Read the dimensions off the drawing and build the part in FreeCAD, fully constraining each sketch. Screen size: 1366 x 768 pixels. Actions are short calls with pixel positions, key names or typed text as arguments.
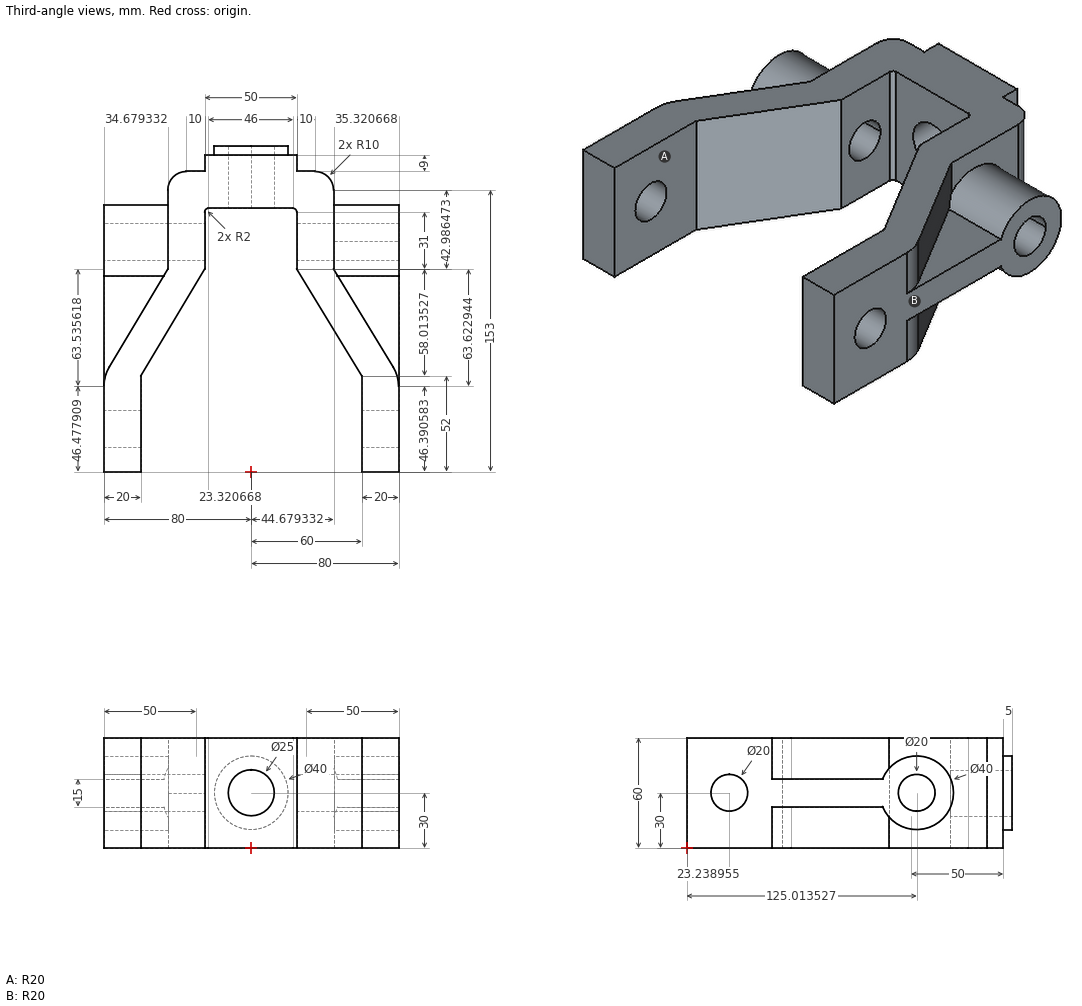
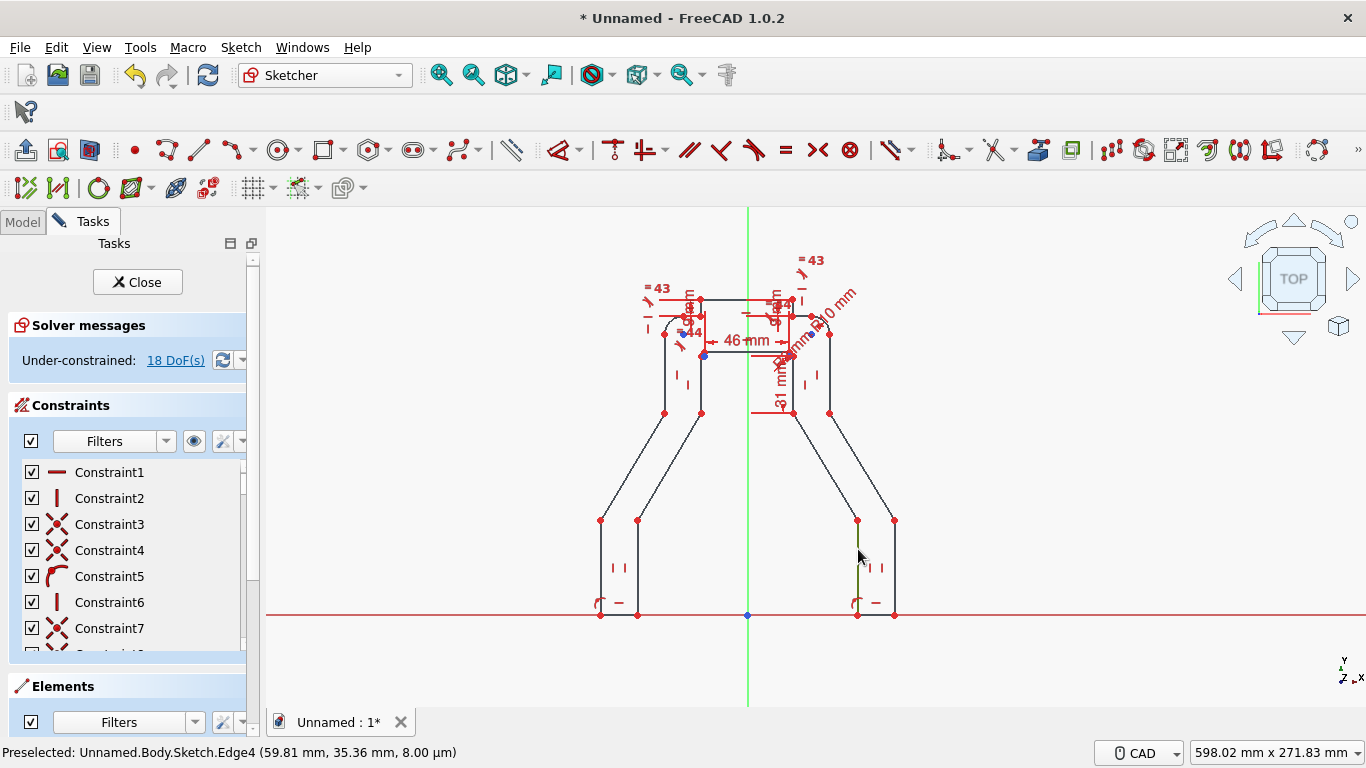
key(i)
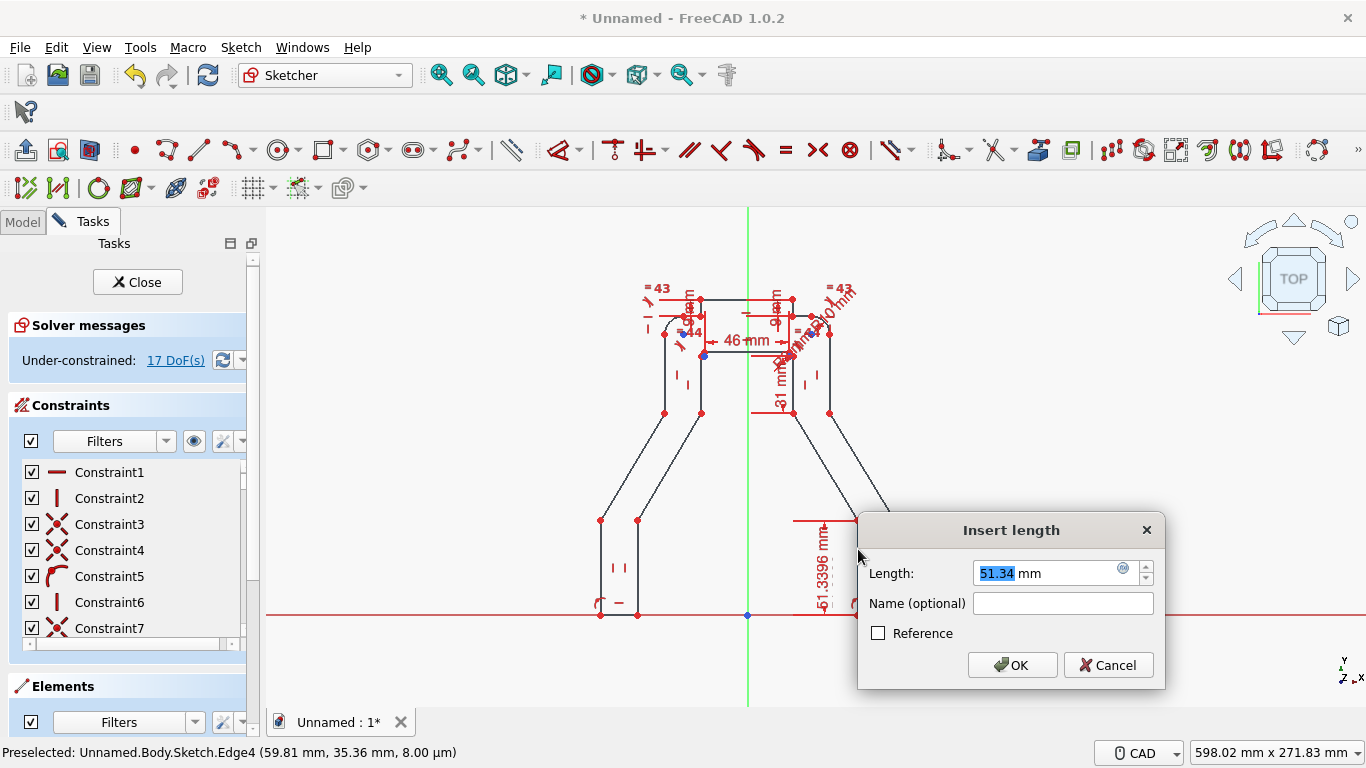
text(52)
key(Return)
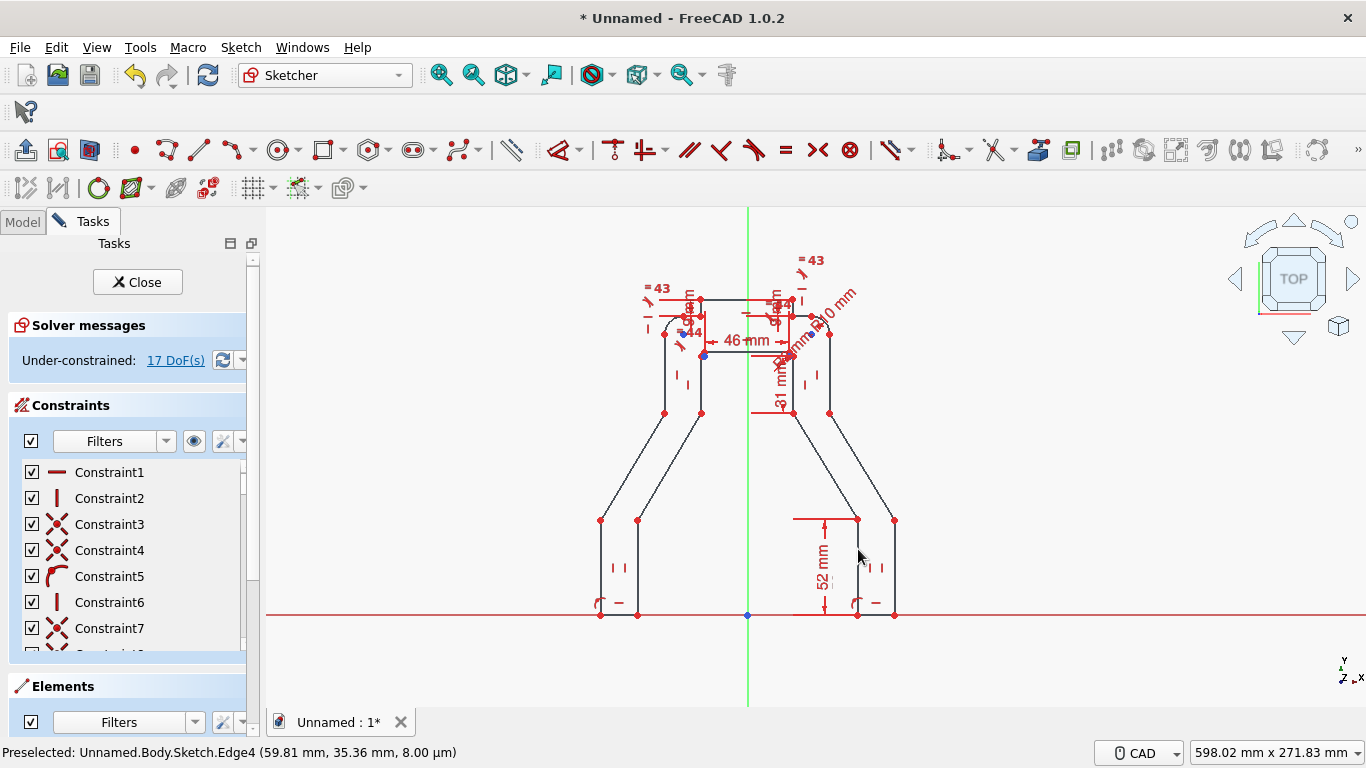
scroll(869, 615, up, 2)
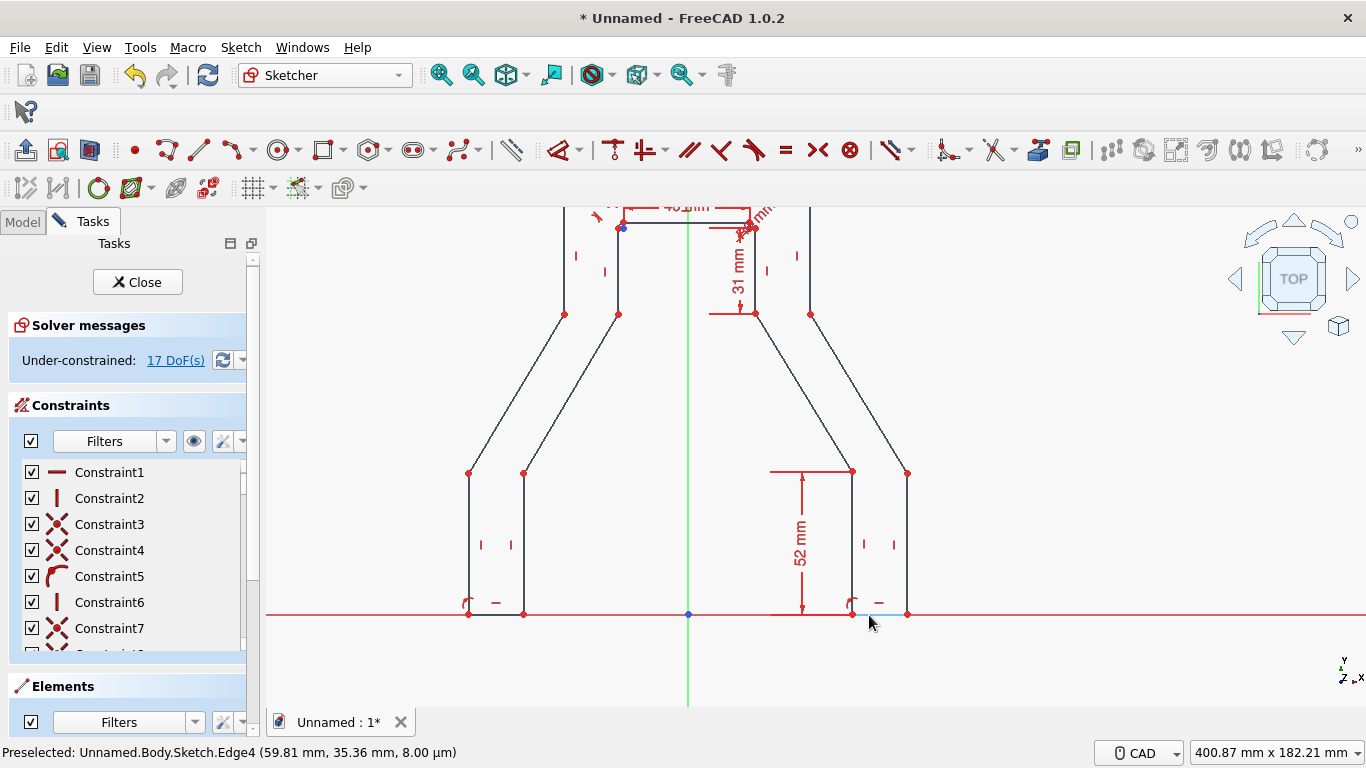
click(869, 615)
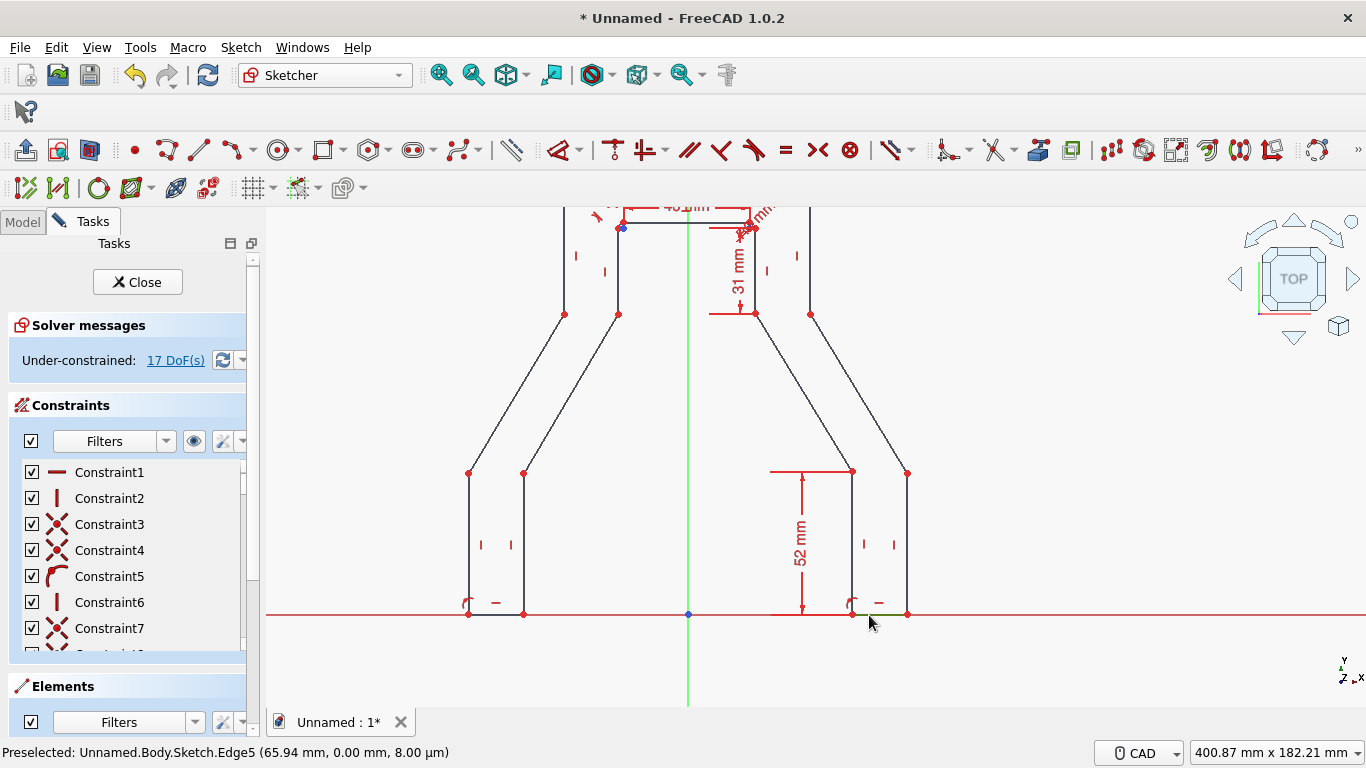
click(582, 150)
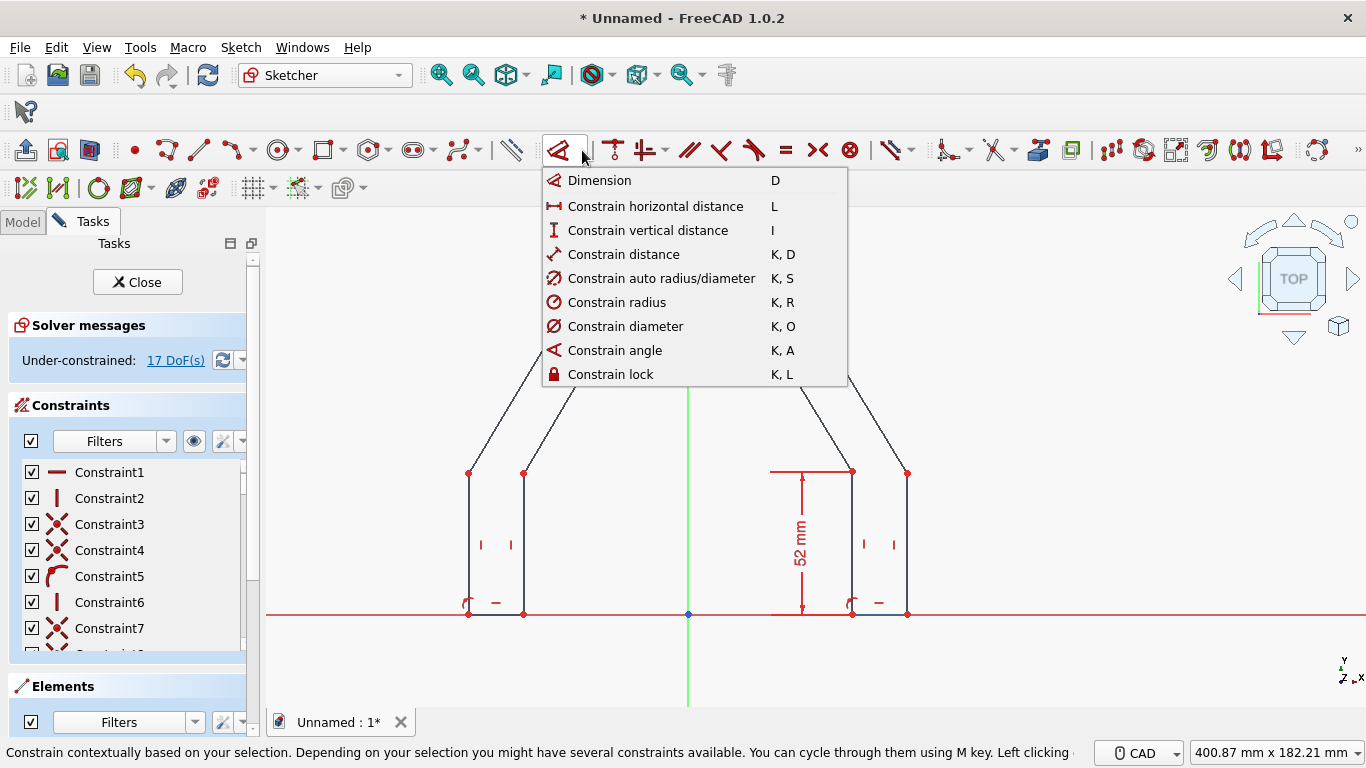
click(695, 206)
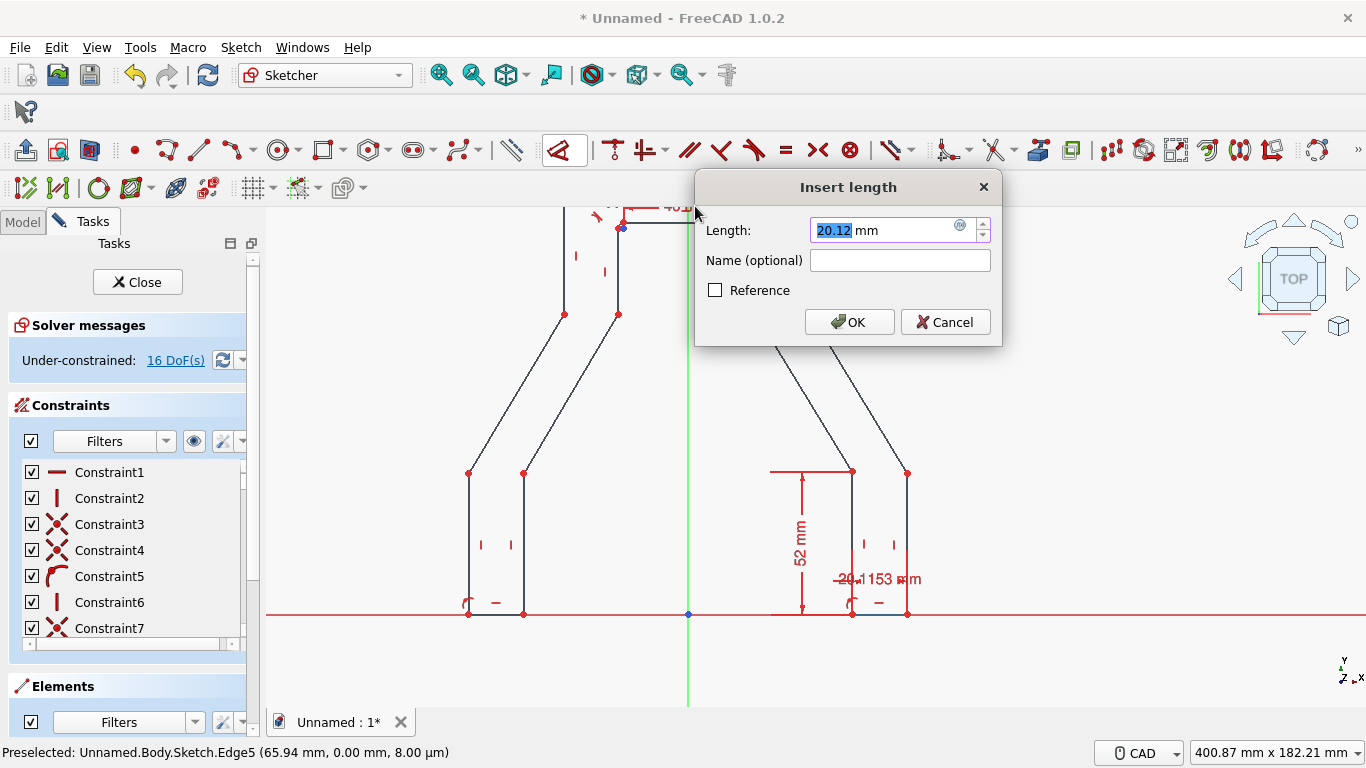
text(20)
key(Return)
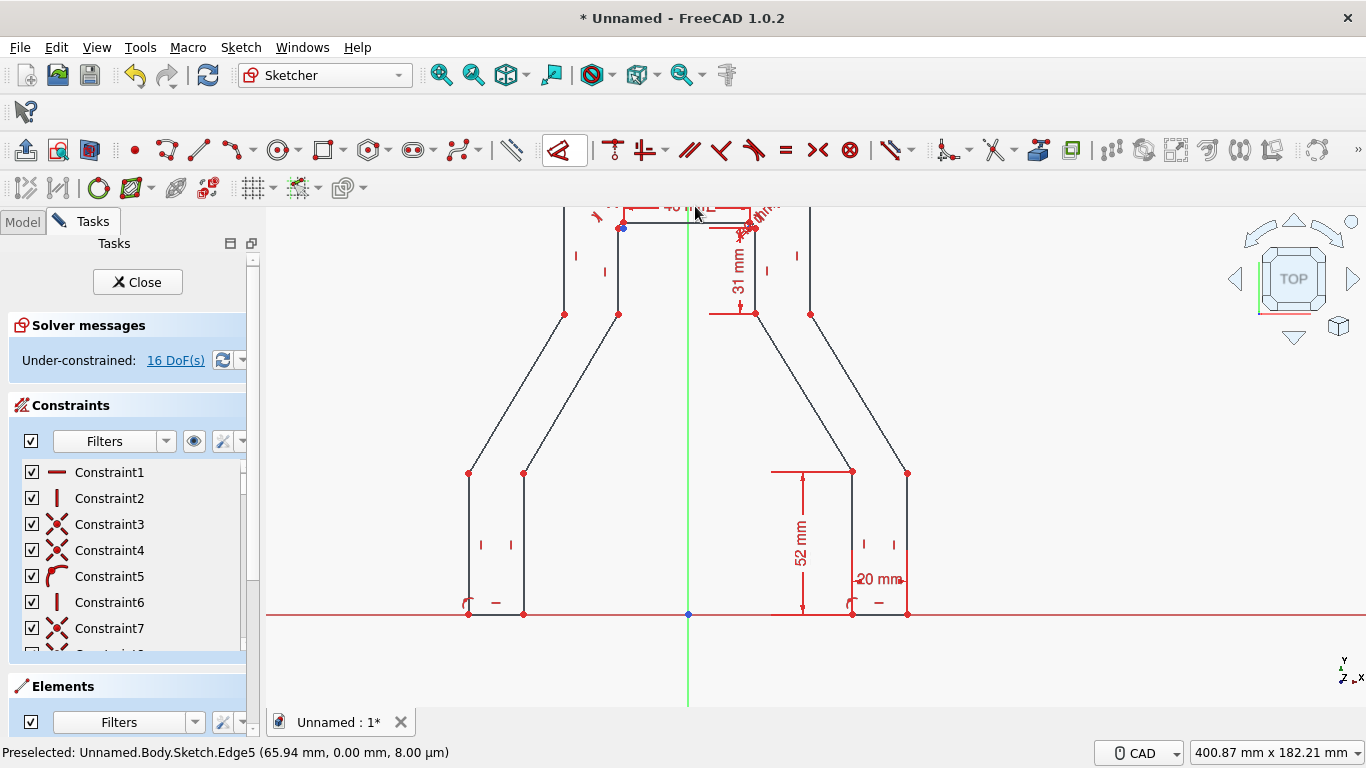
click(907, 572)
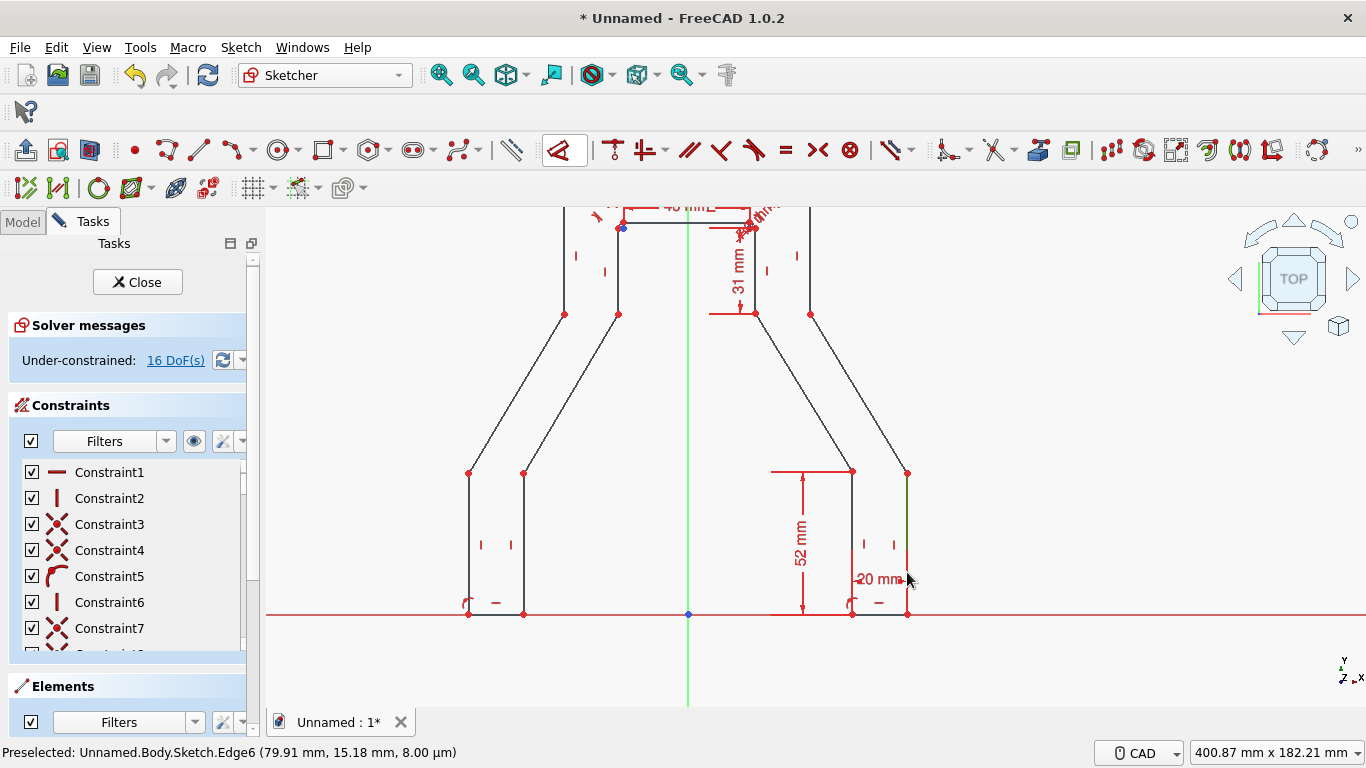
click(582, 150)